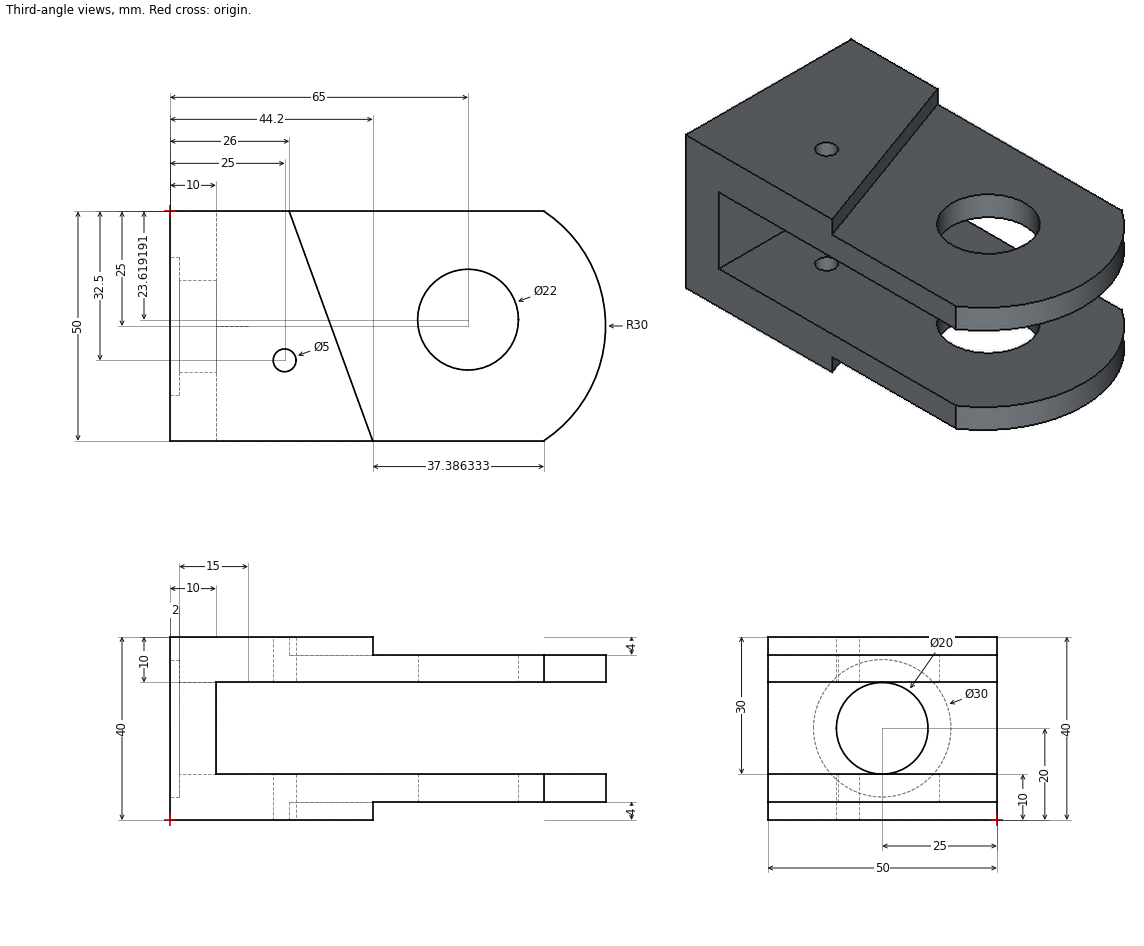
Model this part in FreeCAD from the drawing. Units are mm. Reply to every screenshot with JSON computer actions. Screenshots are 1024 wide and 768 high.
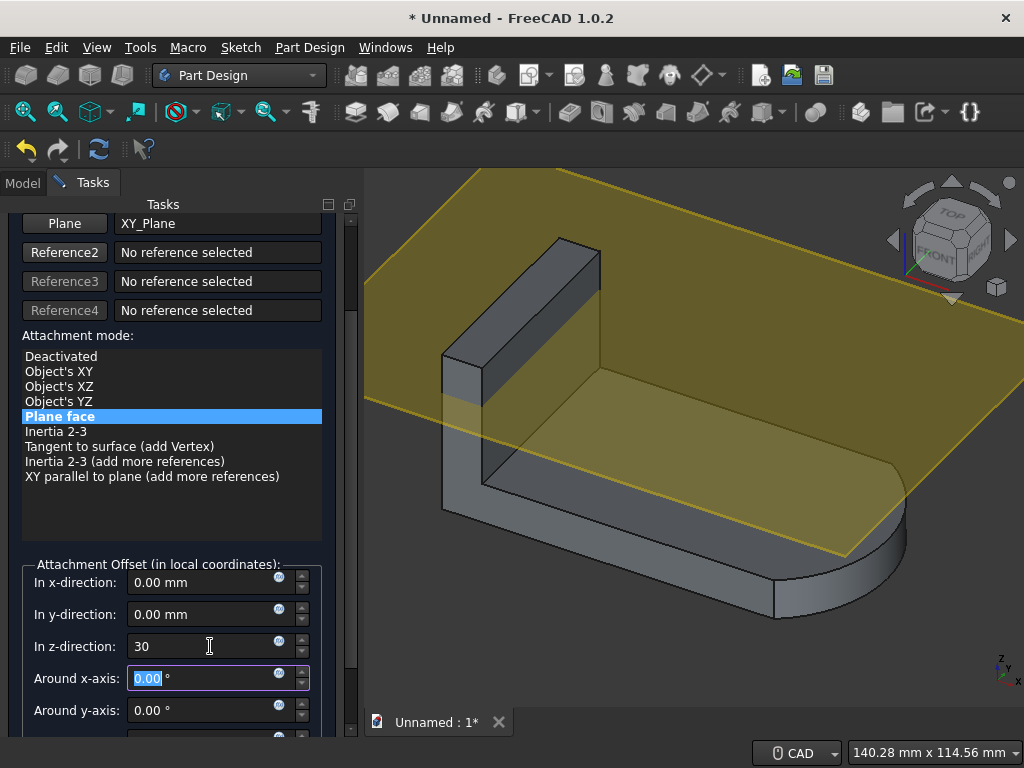
{"action": "scroll", "coordinate": [351, 475], "scroll_direction": "up", "scroll_amount": 3}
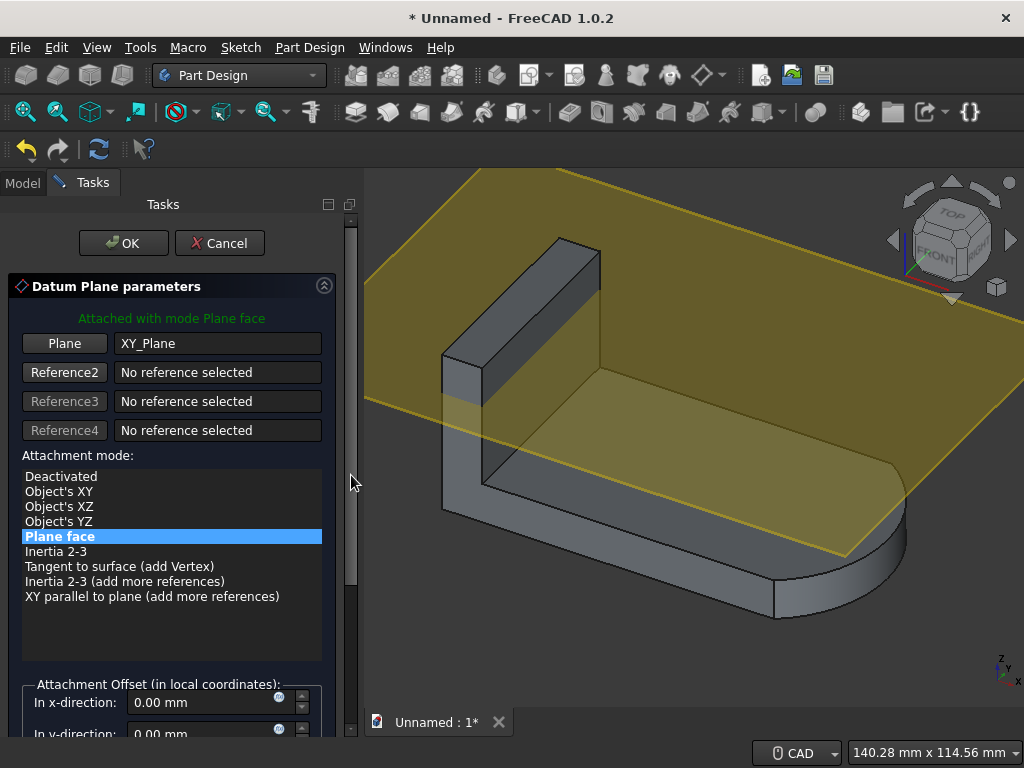
{"action": "left_click", "coordinate": [124, 243]}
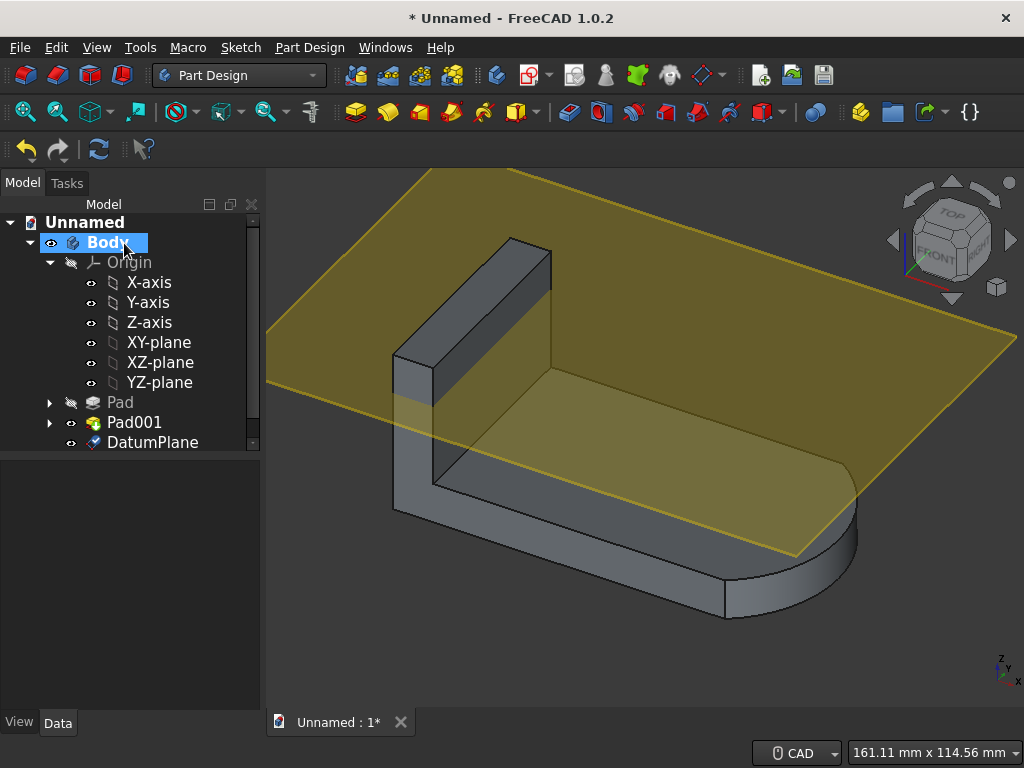
{"action": "left_click", "coordinate": [116, 443]}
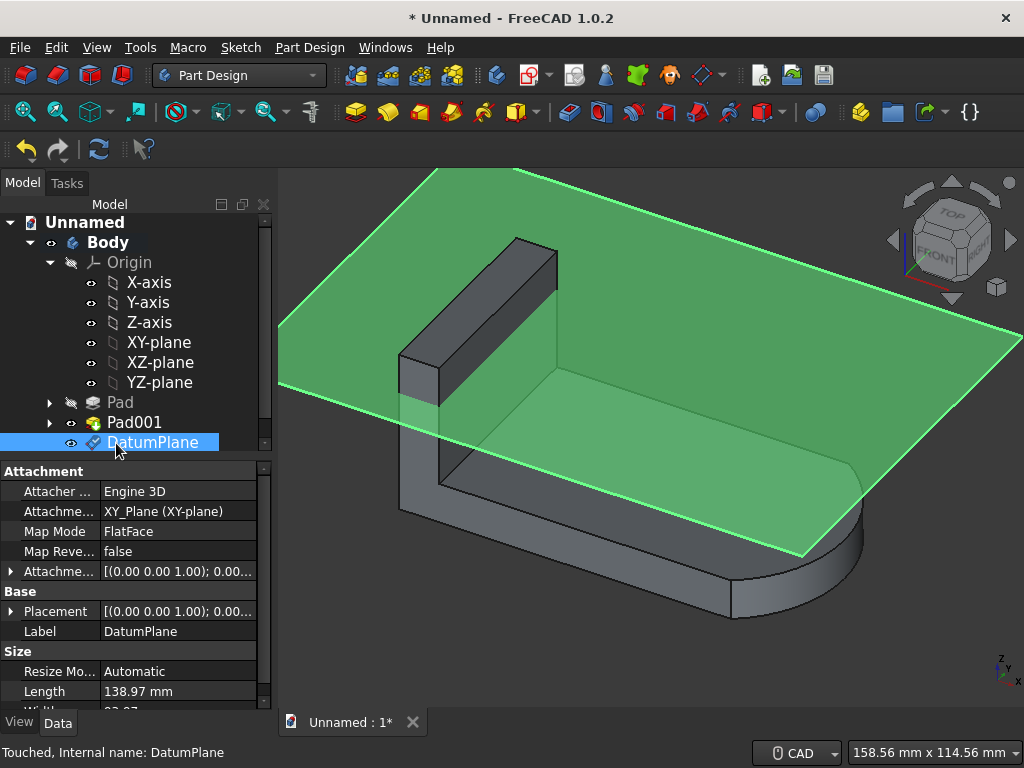
{"action": "left_click", "coordinate": [530, 76]}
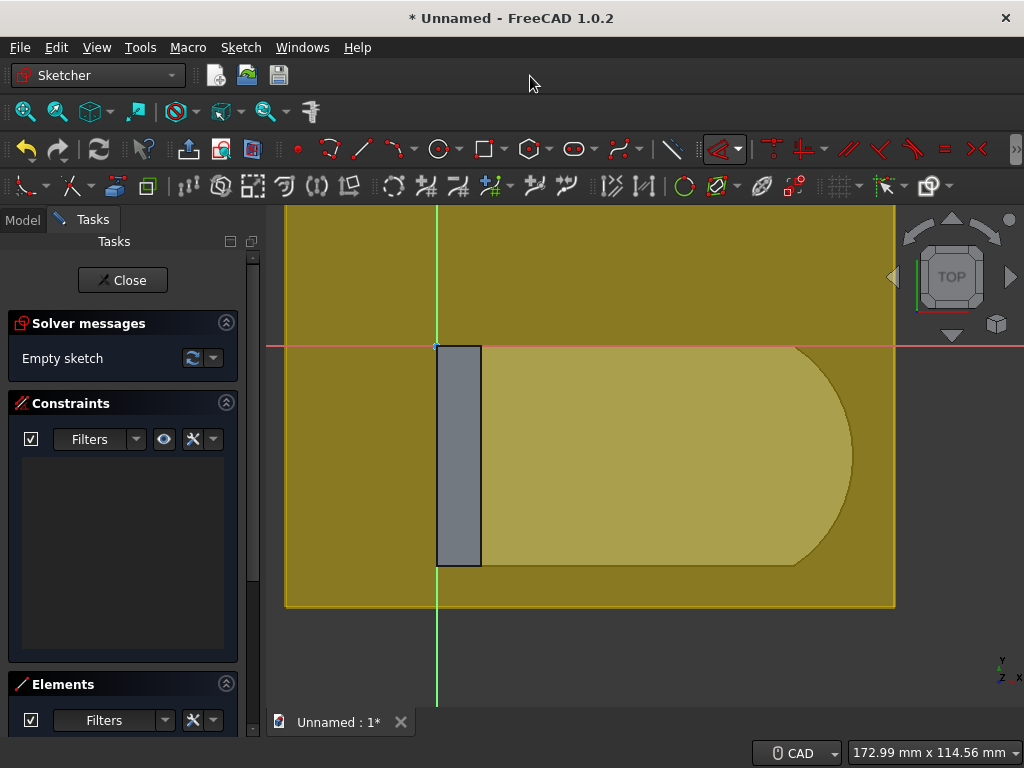
{"action": "left_click", "coordinate": [254, 150]}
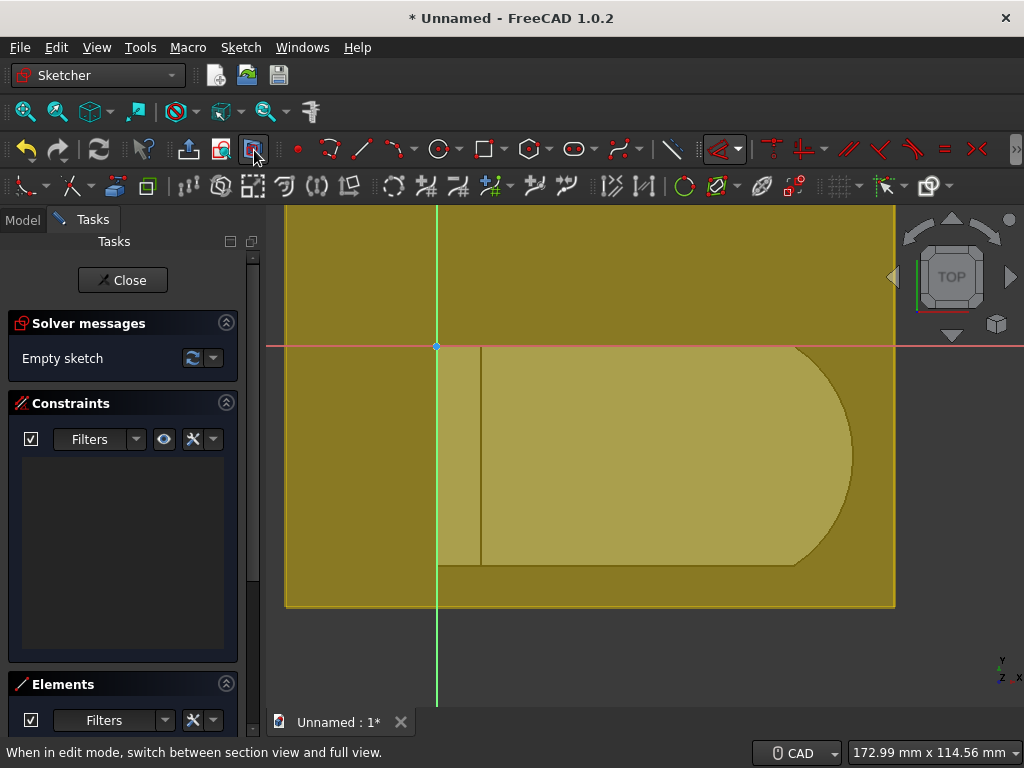
{"action": "scroll", "coordinate": [294, 456], "scroll_direction": "down", "scroll_amount": 1}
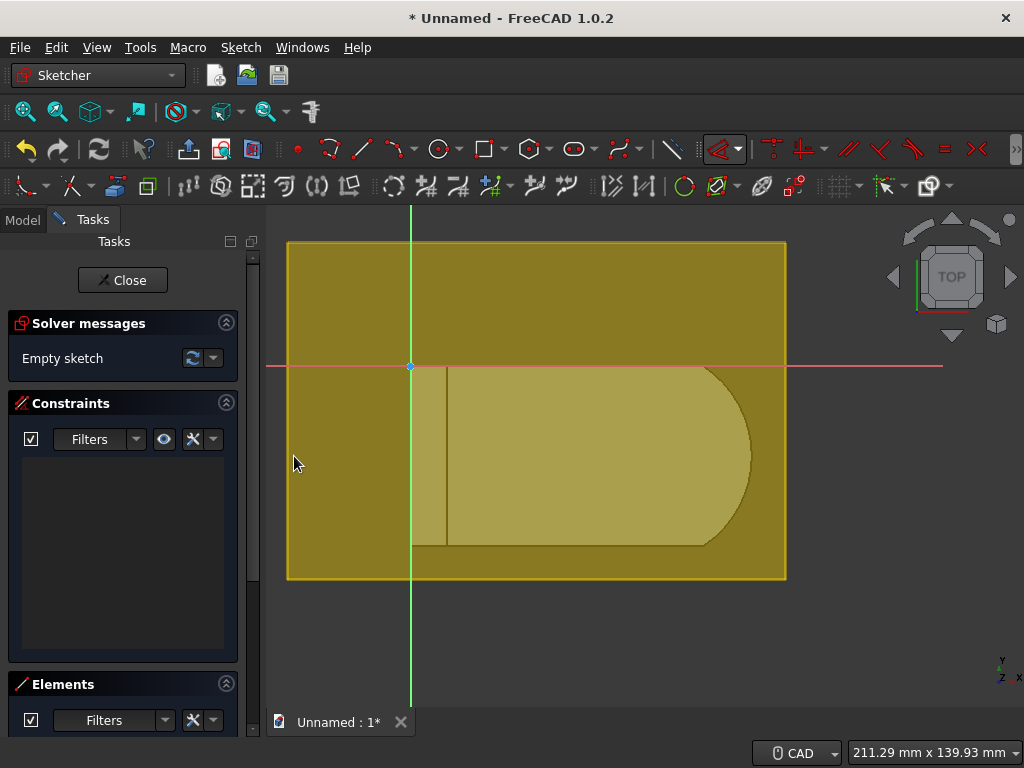
{"action": "left_click", "coordinate": [330, 150]}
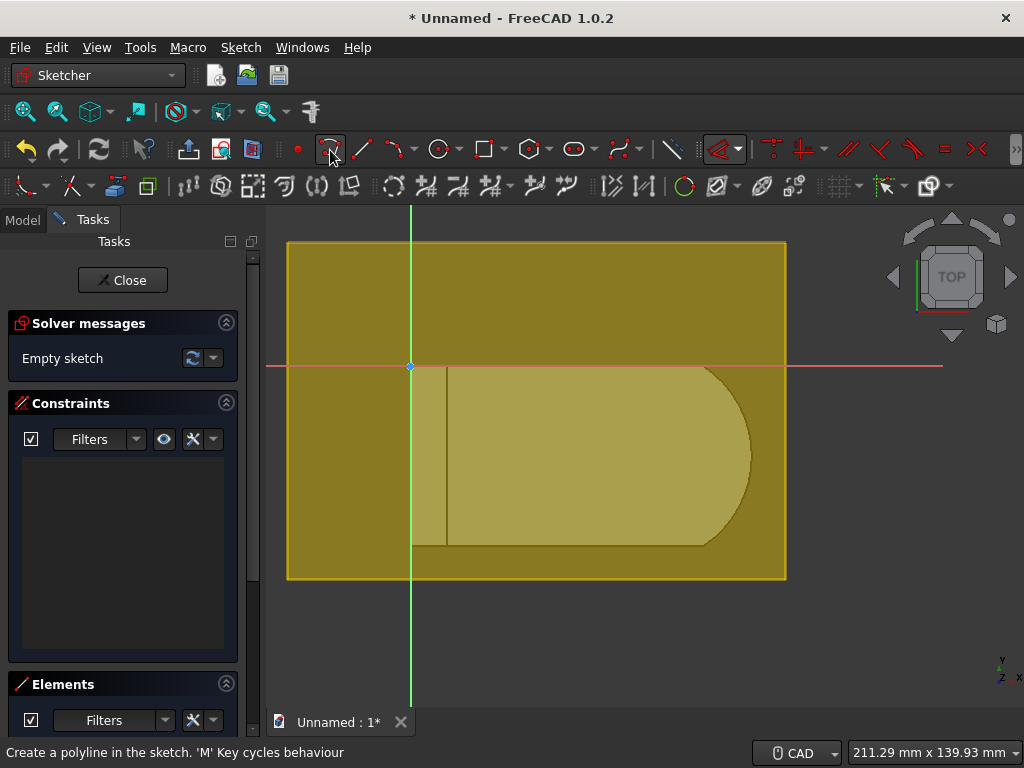
{"action": "left_click", "coordinate": [704, 366]}
{"action": "left_click", "coordinate": [447, 375]}
{"action": "left_click", "coordinate": [447, 546]}
{"action": "left_click", "coordinate": [704, 546]}
{"action": "right_click", "coordinate": [704, 546]}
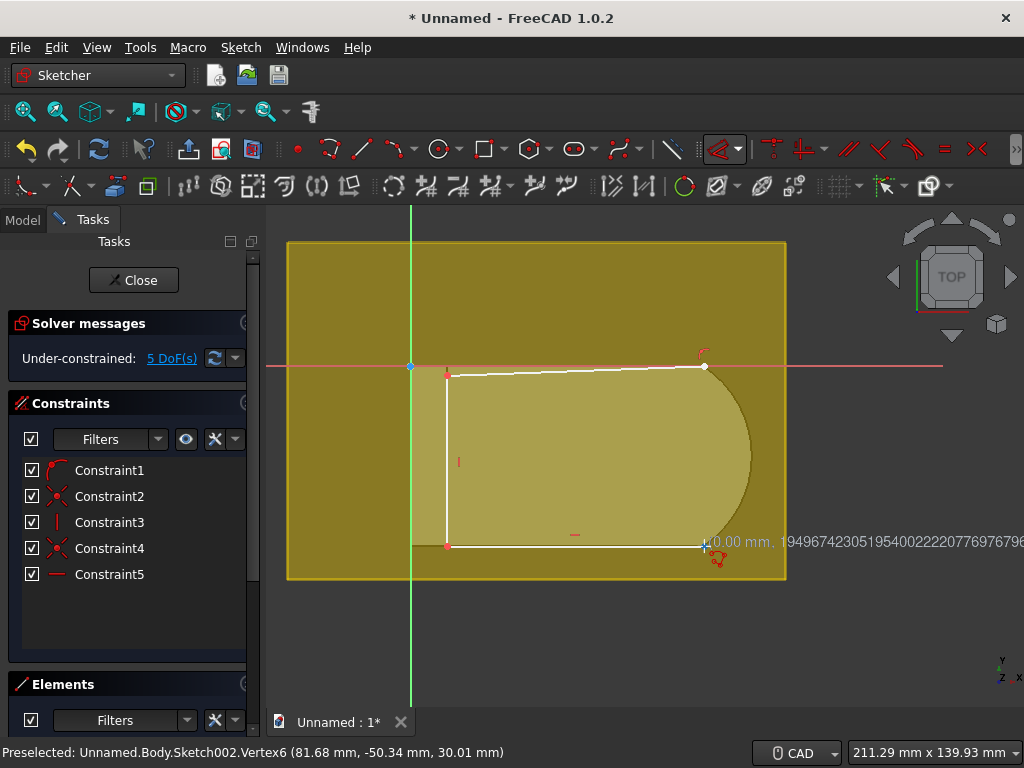
{"action": "left_click", "coordinate": [394, 150]}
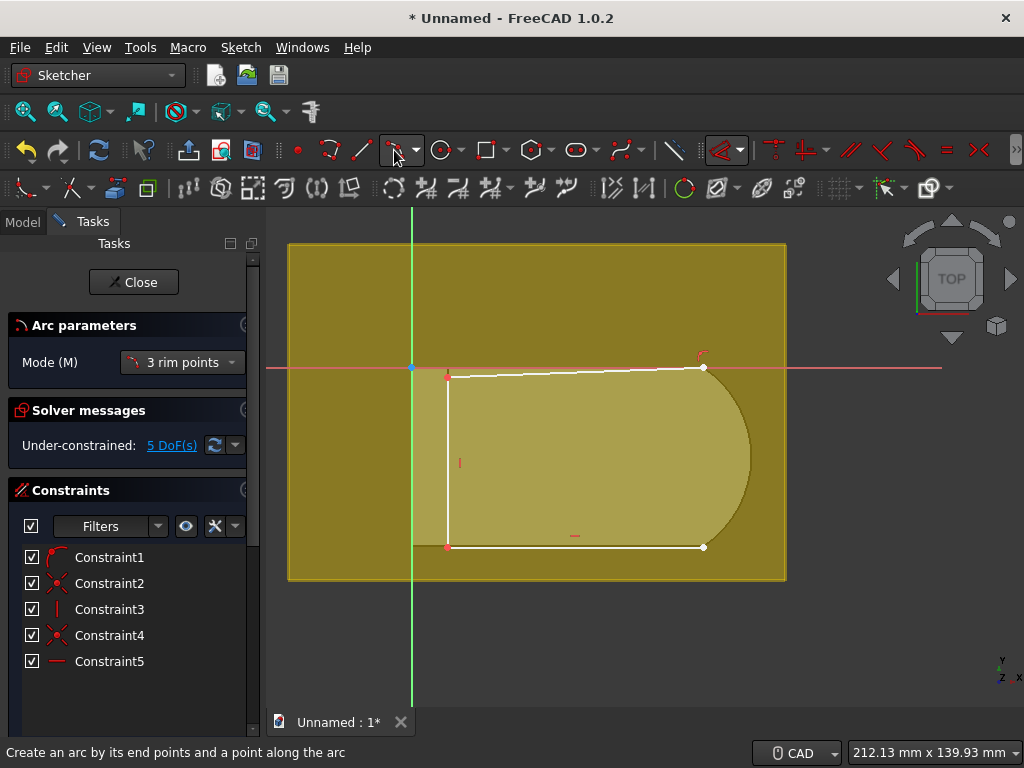
{"action": "left_click", "coordinate": [704, 548]}
{"action": "left_click", "coordinate": [704, 368]}
{"action": "left_click", "coordinate": [751, 457]}
{"action": "key", "text": "Escape"}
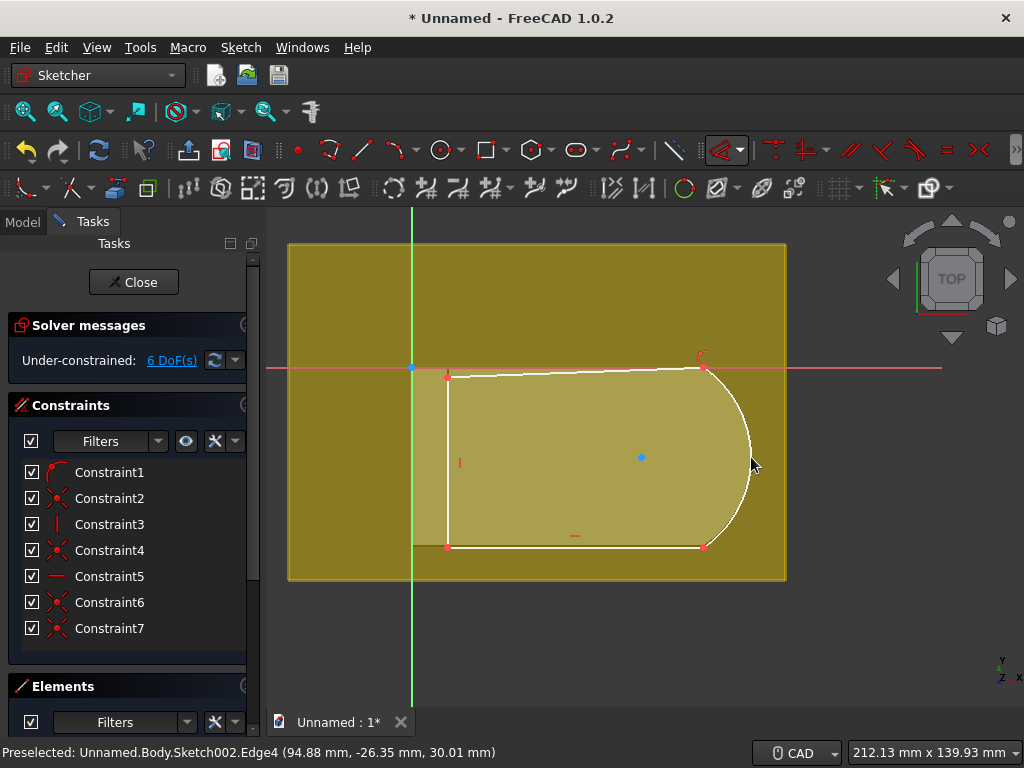
{"action": "left_click", "coordinate": [627, 371]}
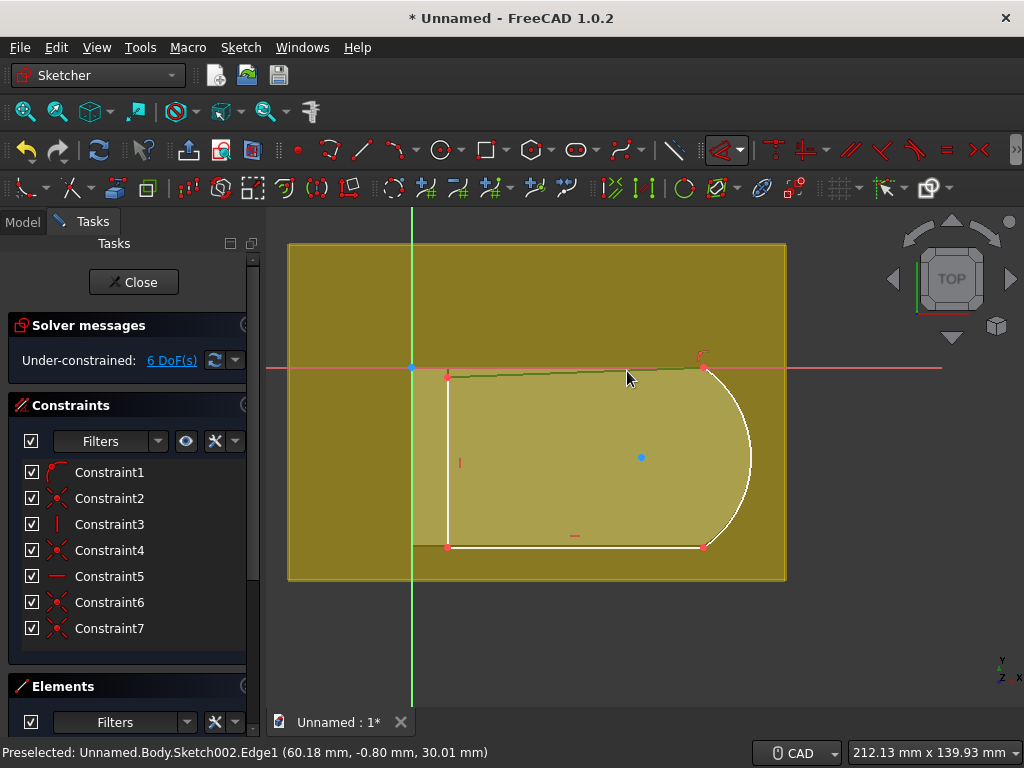
{"action": "key", "text": "h"}